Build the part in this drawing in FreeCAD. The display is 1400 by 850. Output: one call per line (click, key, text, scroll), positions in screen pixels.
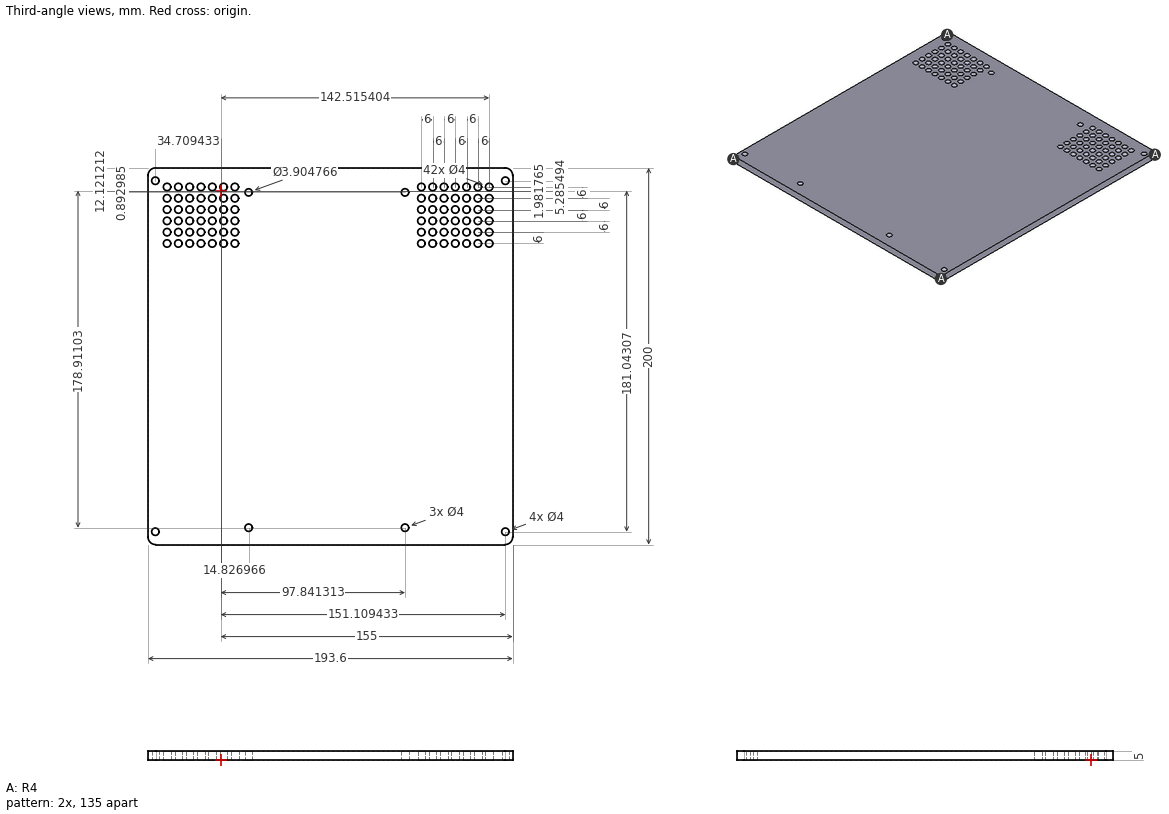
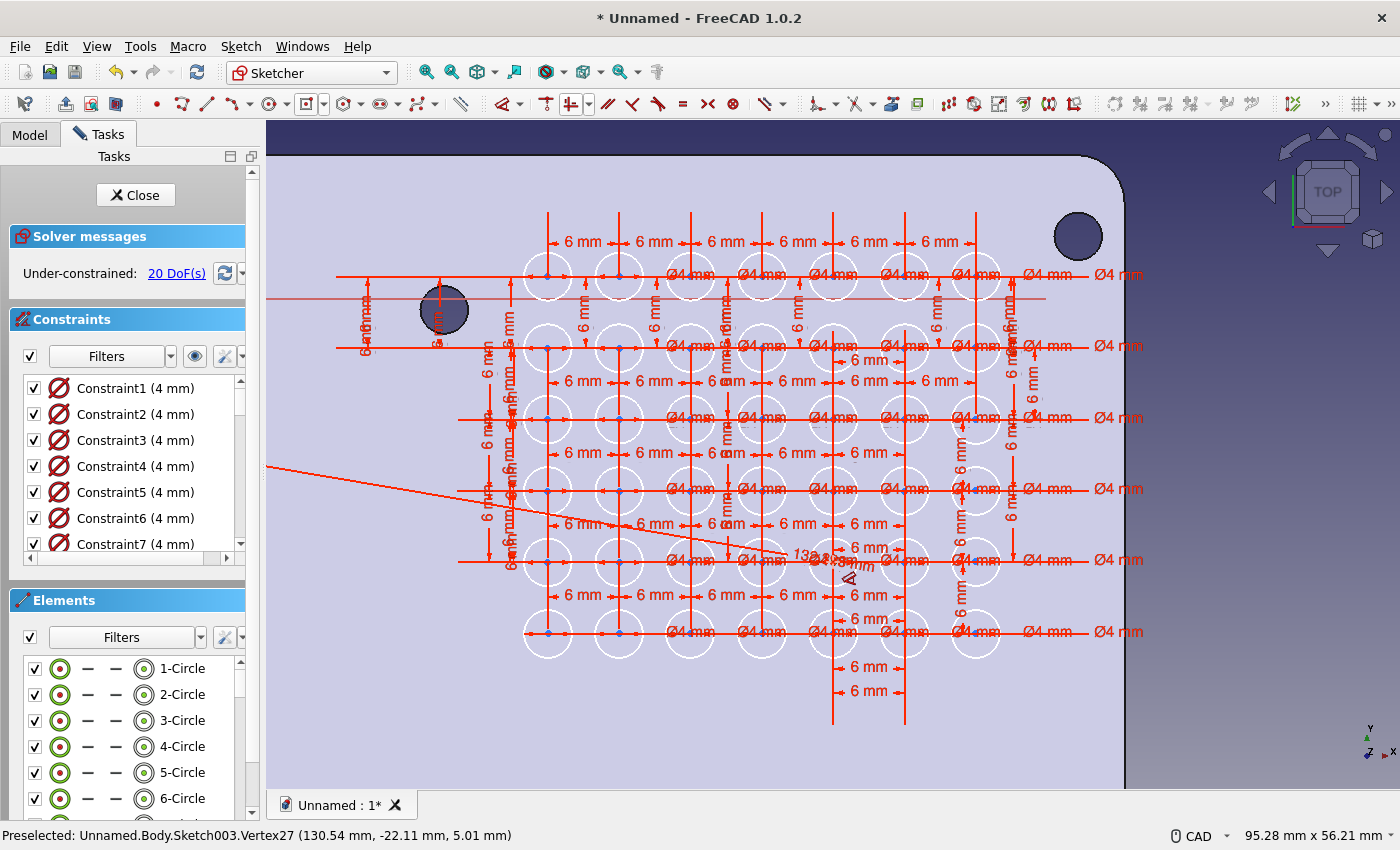
click(833, 634)
click(1013, 573)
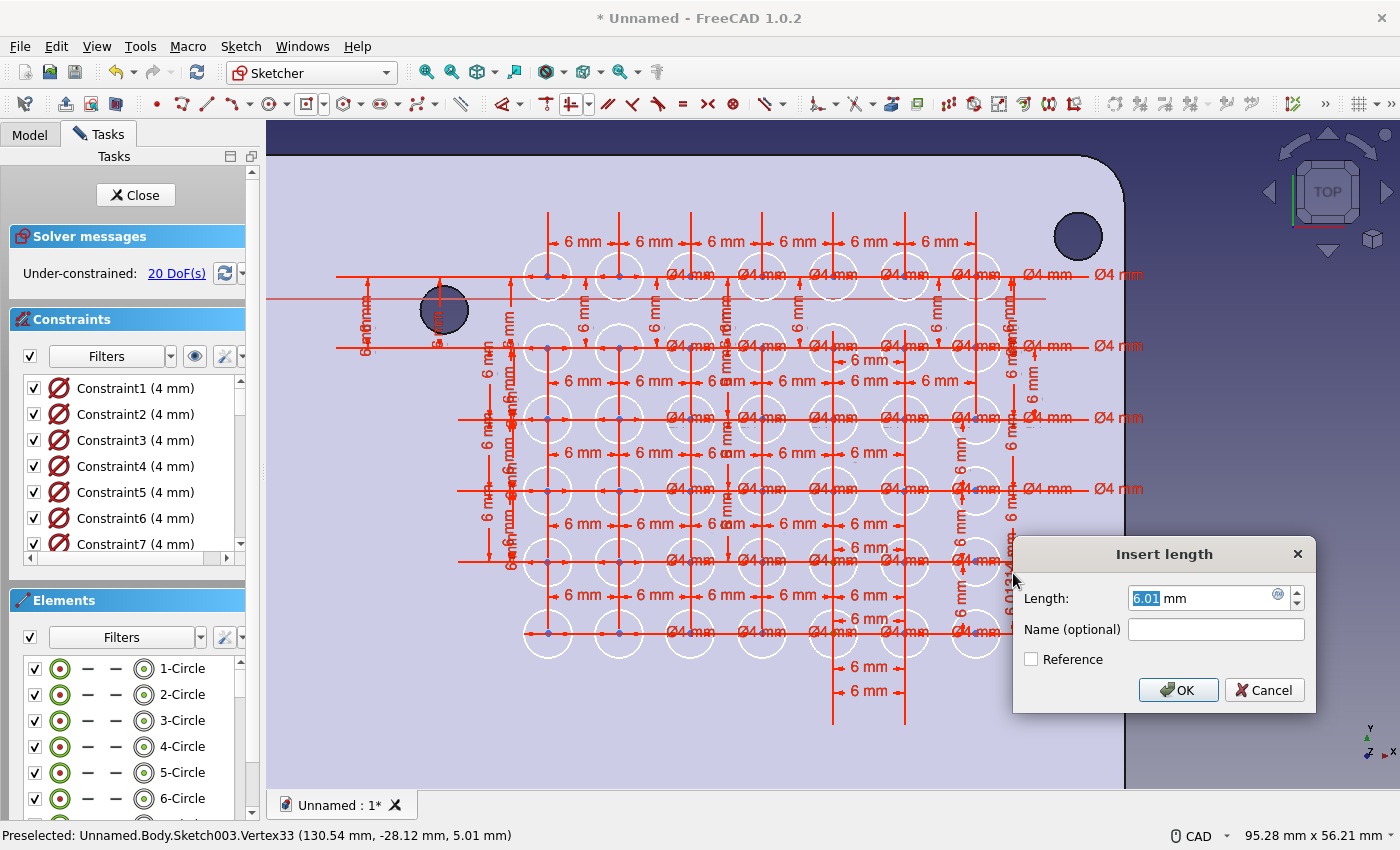
text(6)
key(Return)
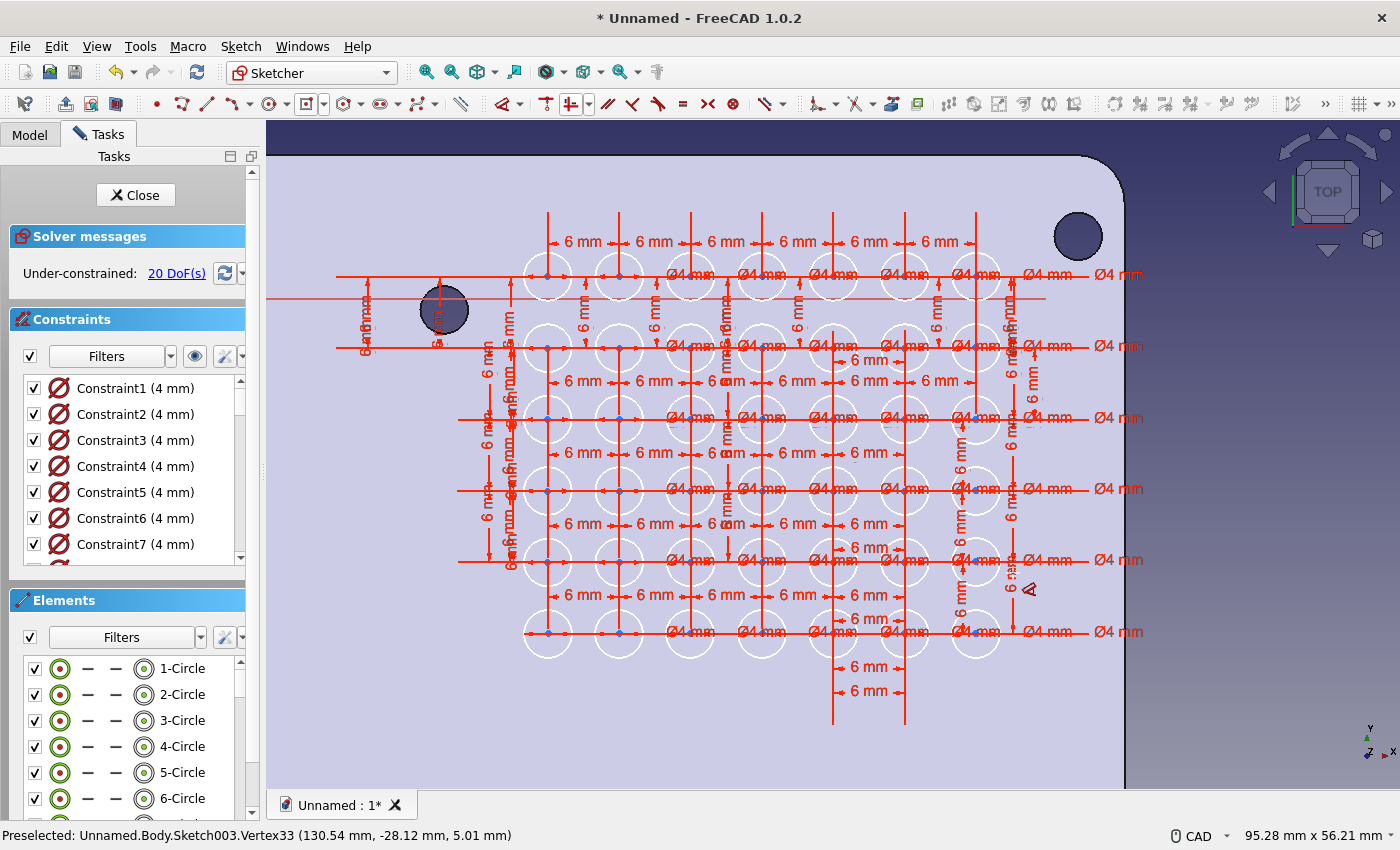
click(833, 634)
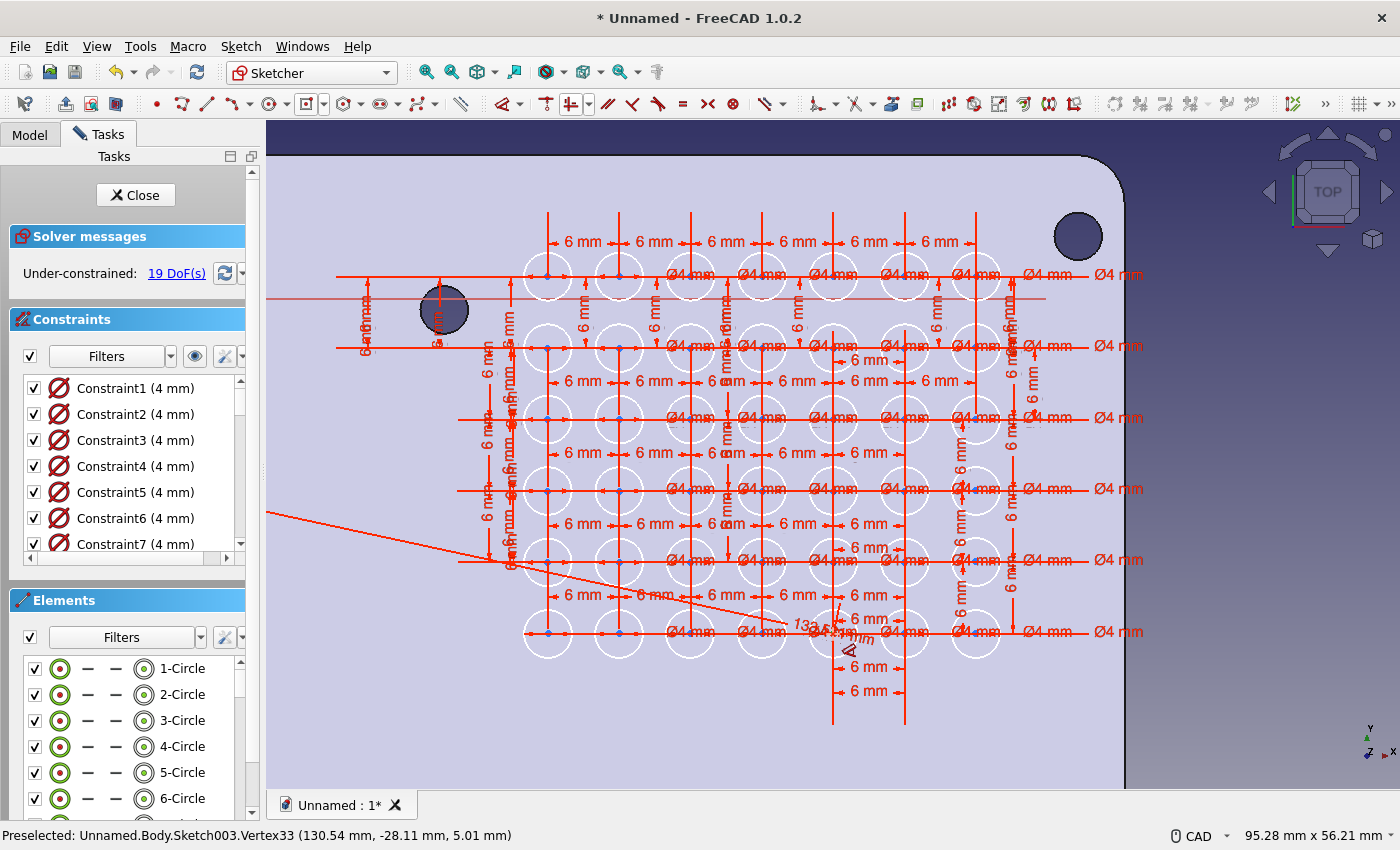
click(762, 634)
click(798, 668)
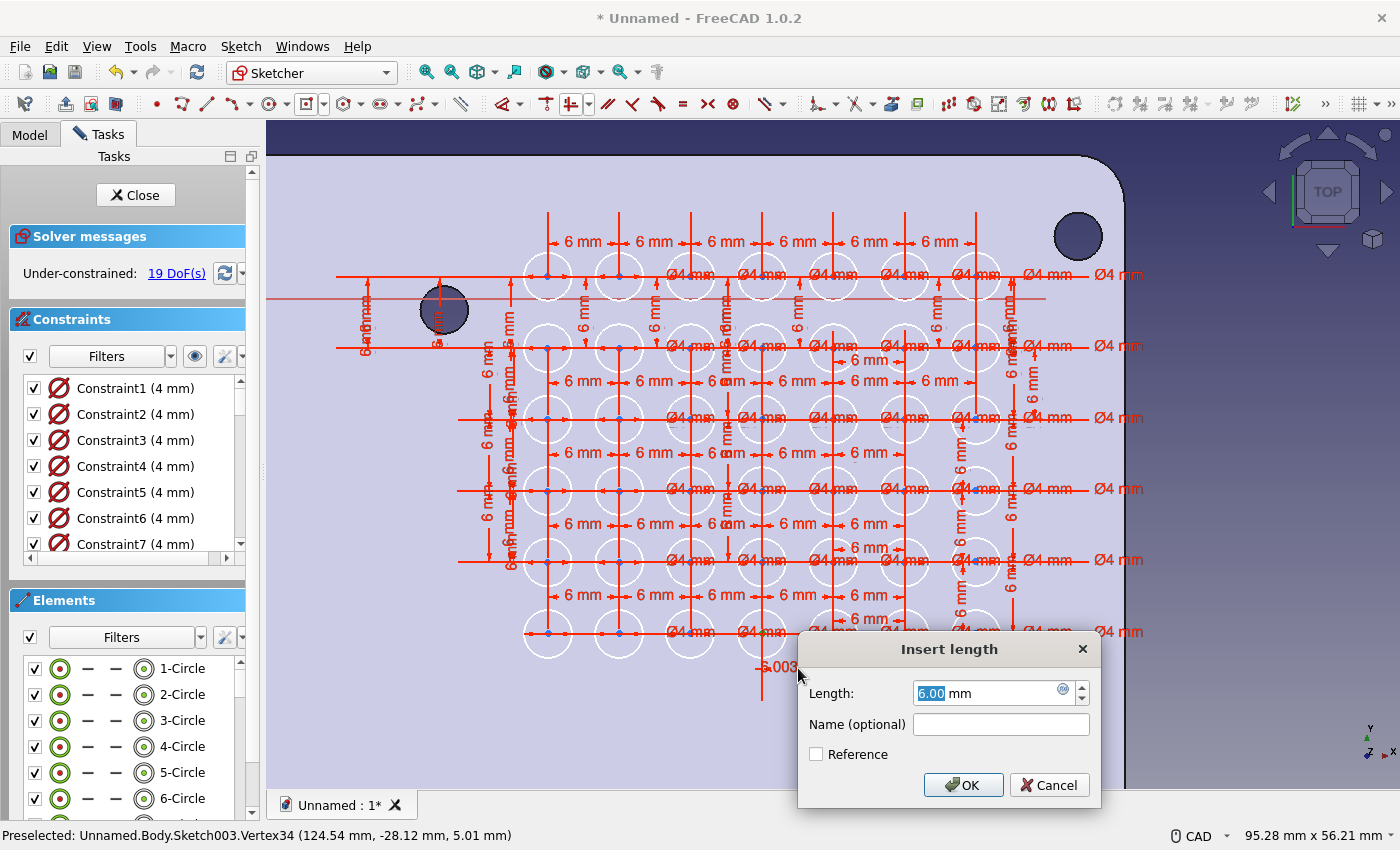
text(6)
key(Return)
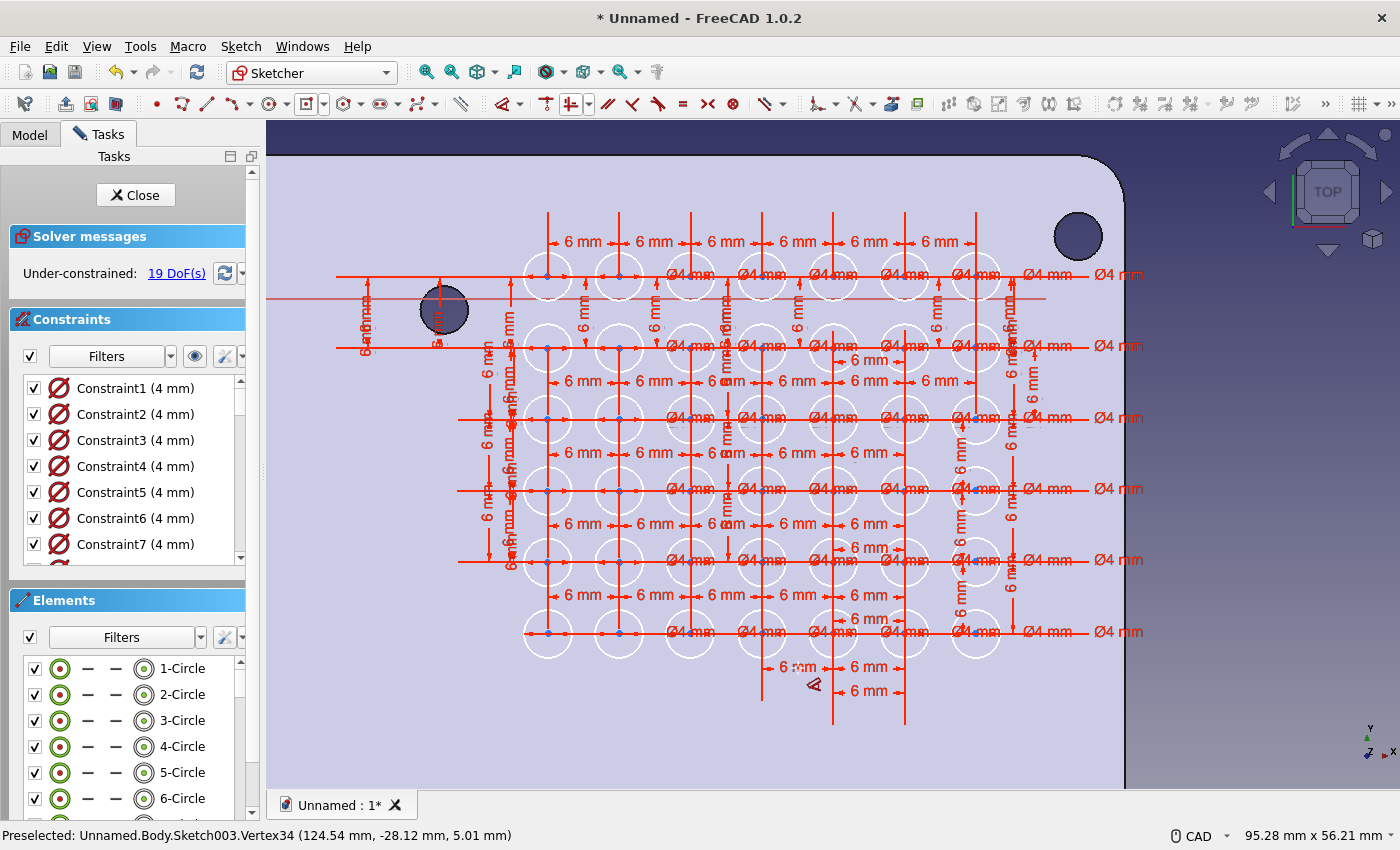
click(762, 562)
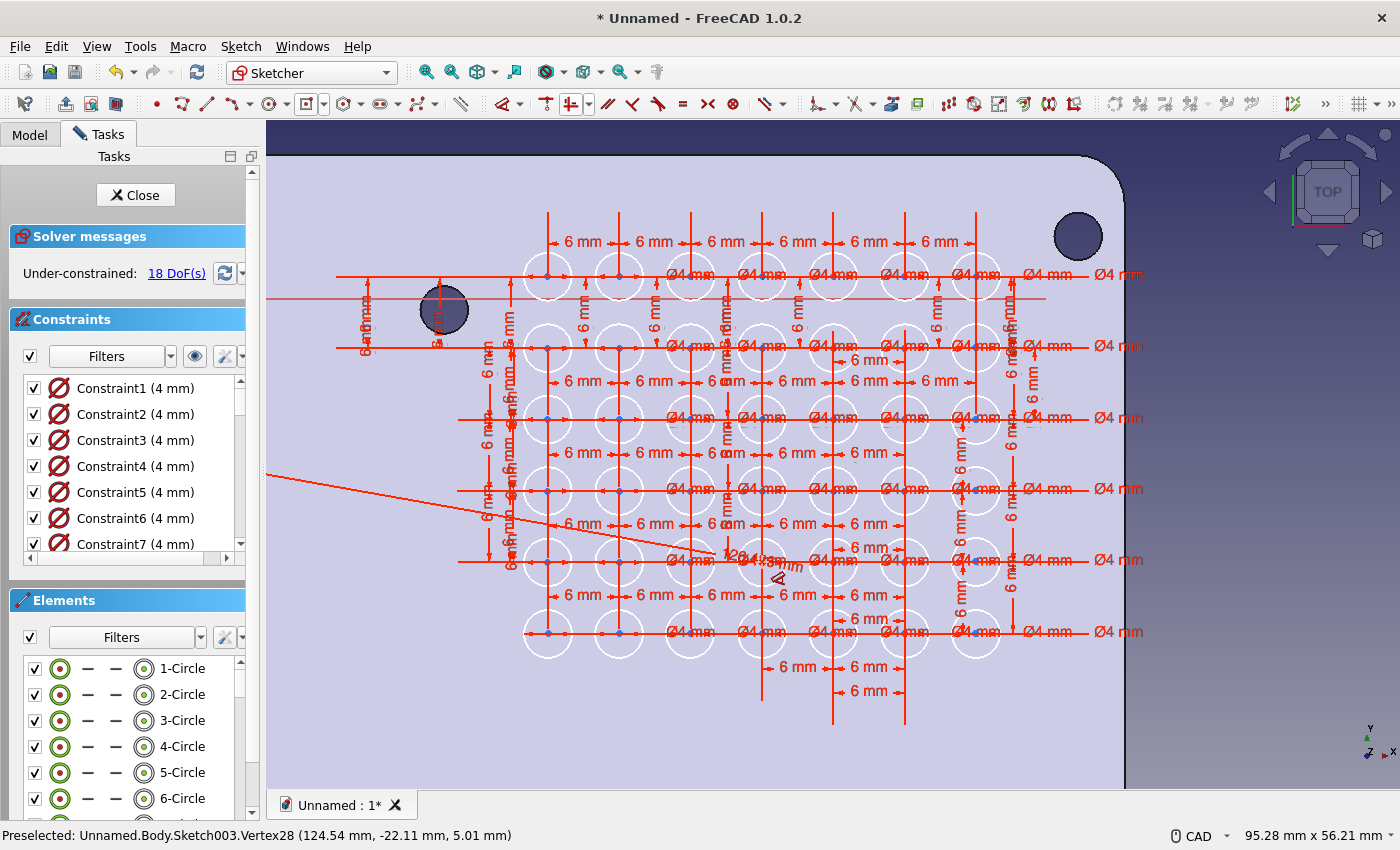
click(762, 634)
click(796, 582)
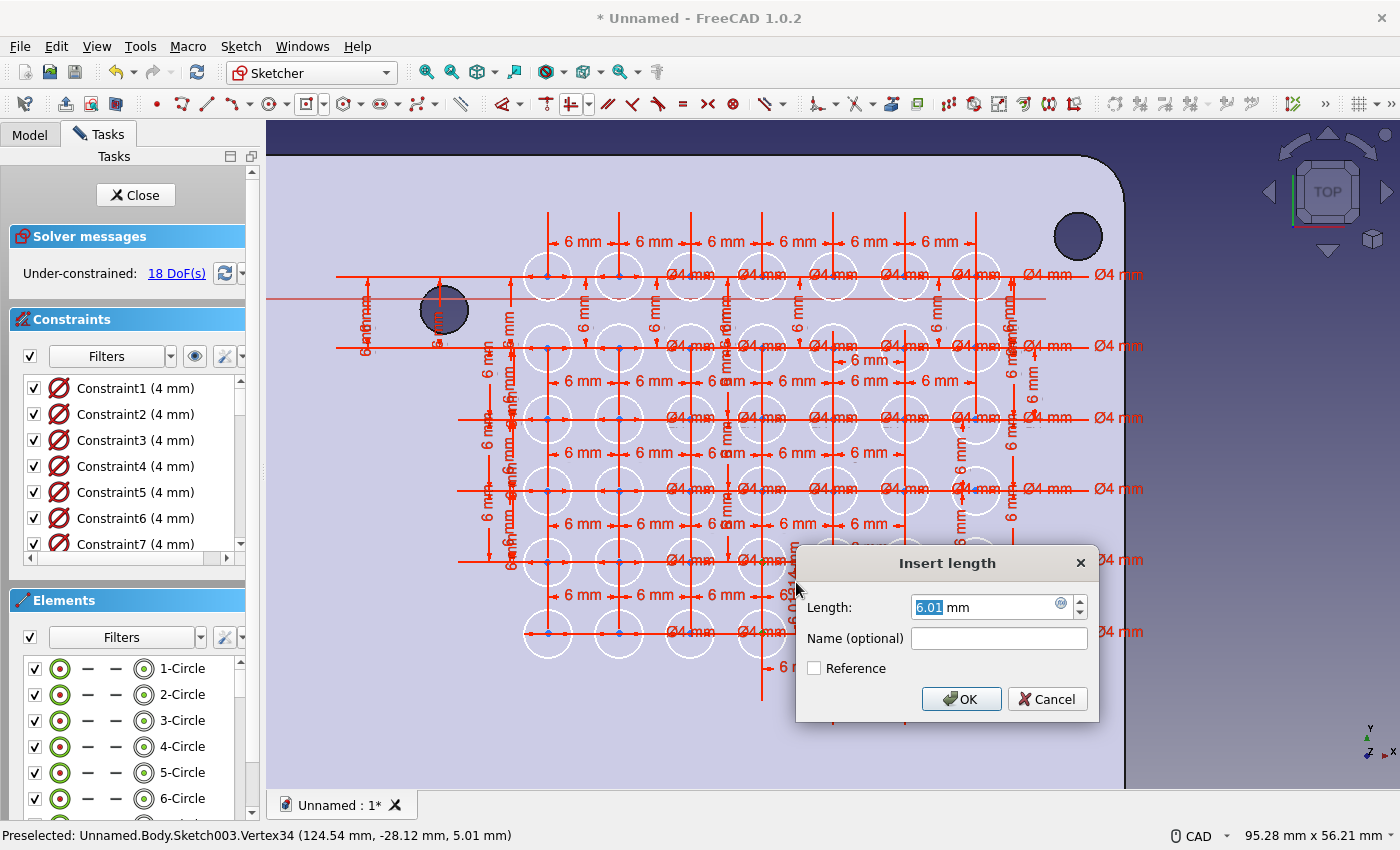
text(6)
key(Return)